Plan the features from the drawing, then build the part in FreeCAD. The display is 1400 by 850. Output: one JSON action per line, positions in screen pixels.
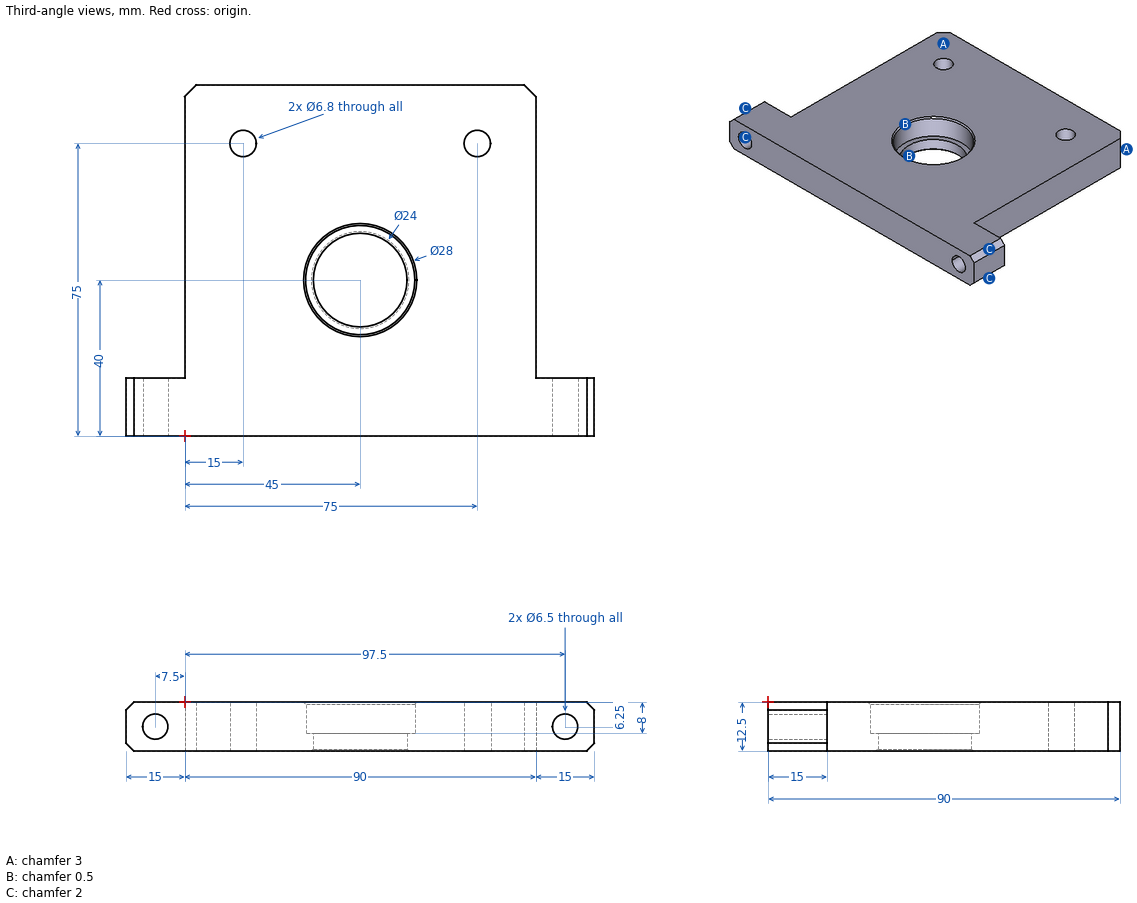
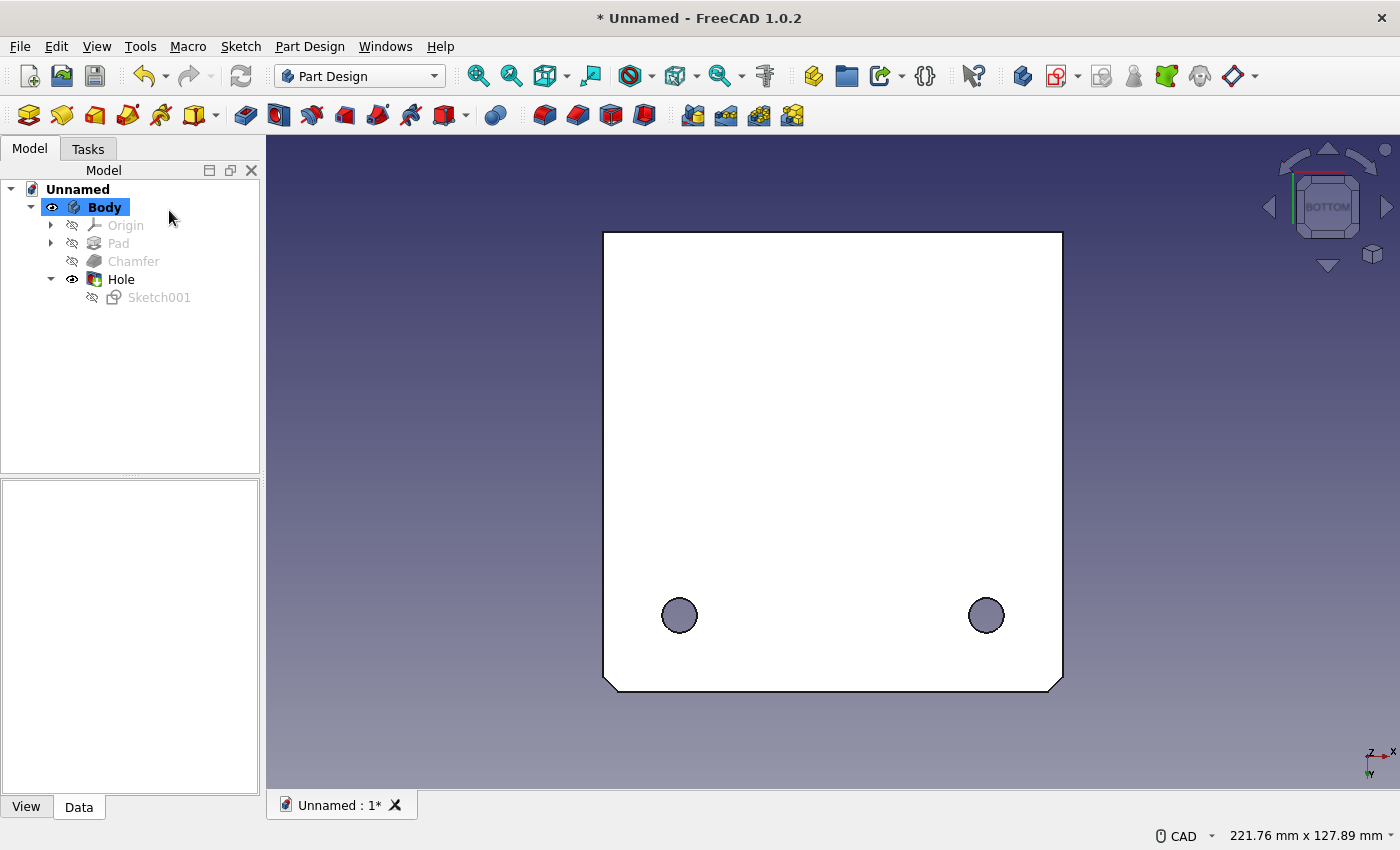
{"action": "left_click", "coordinate": [1056, 76]}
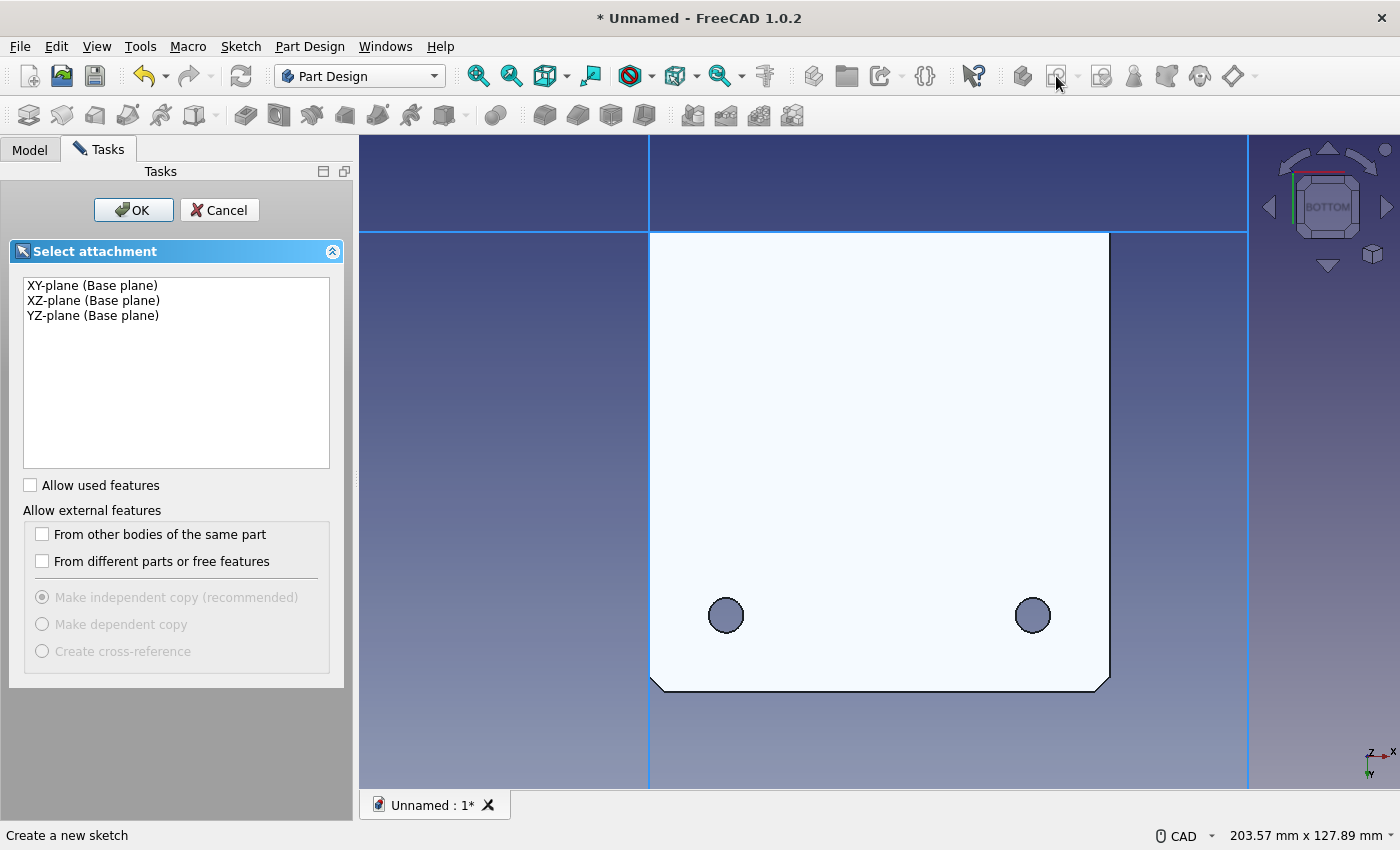
{"action": "left_click", "coordinate": [84, 286]}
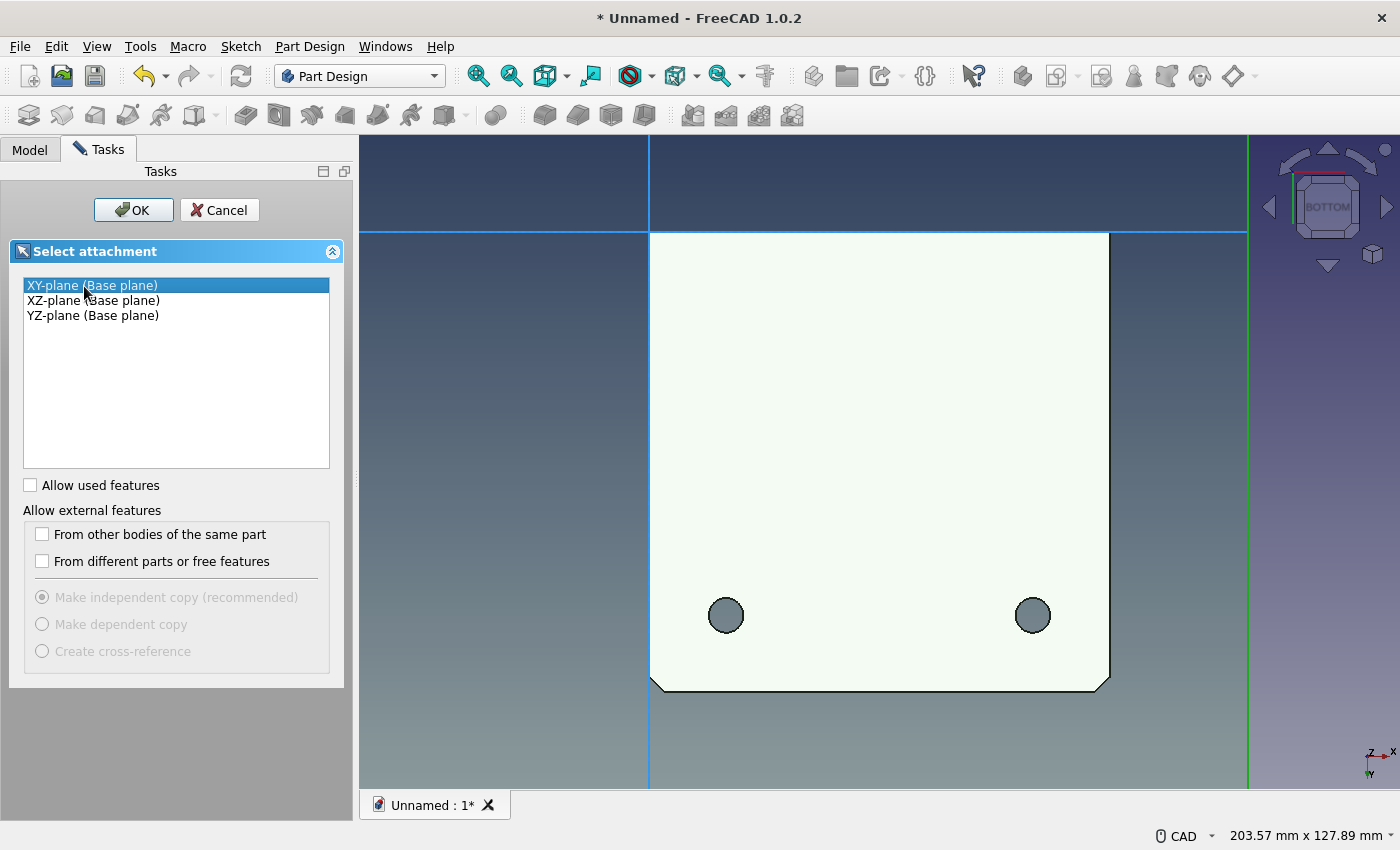
{"action": "left_click", "coordinate": [134, 210]}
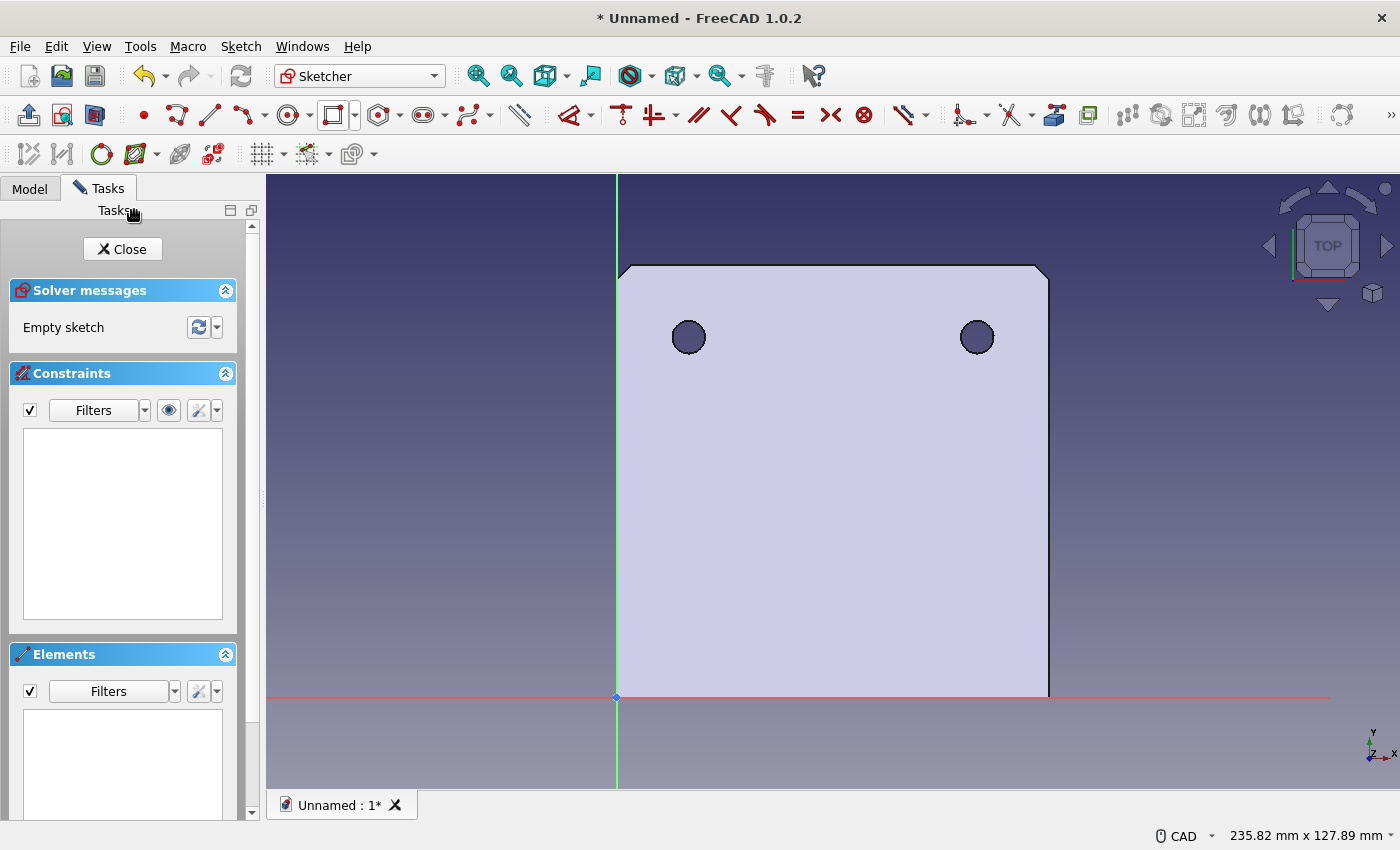
{"action": "scroll", "coordinate": [746, 744], "scroll_direction": "up", "scroll_amount": 2}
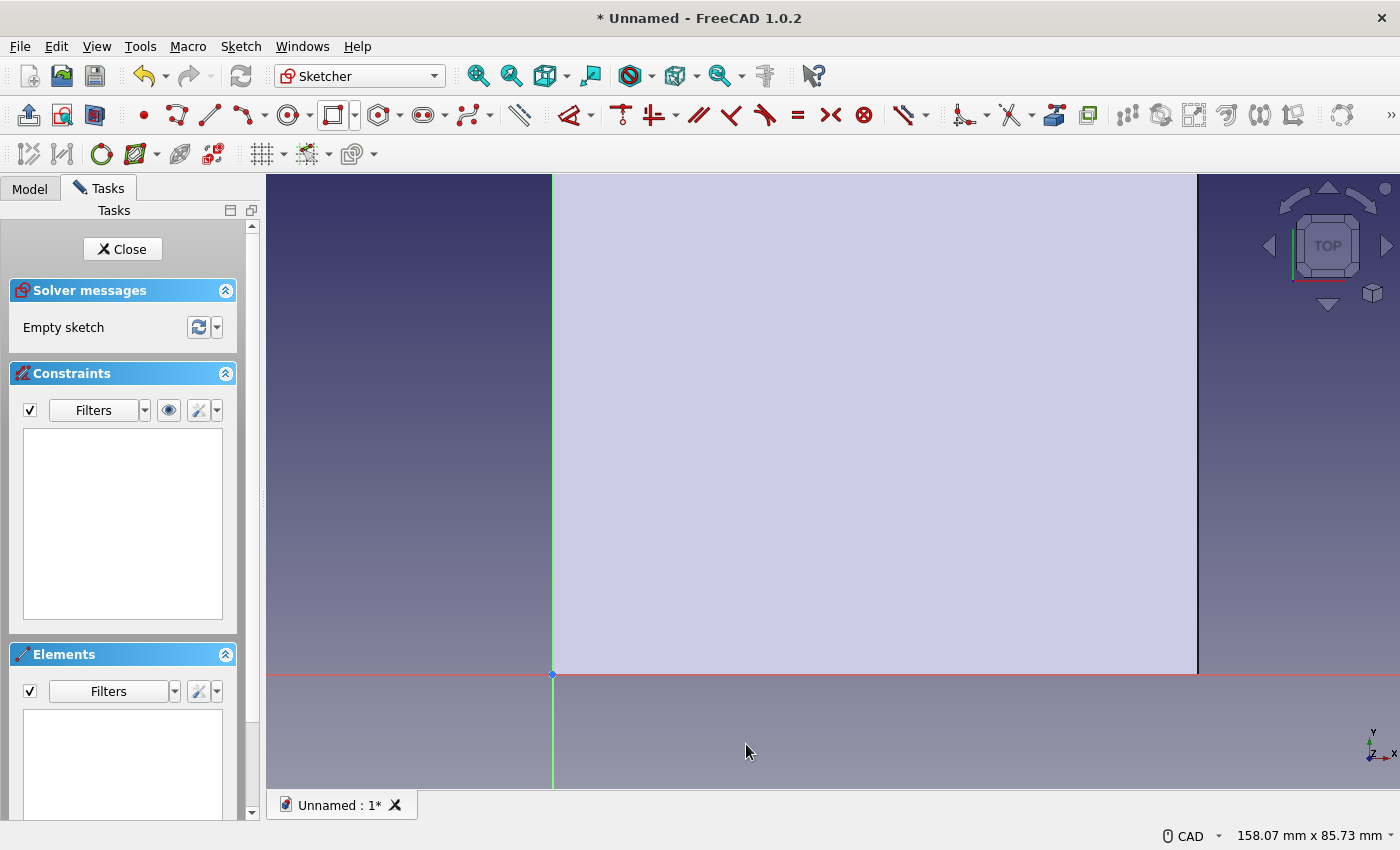
{"action": "left_click", "coordinate": [288, 116]}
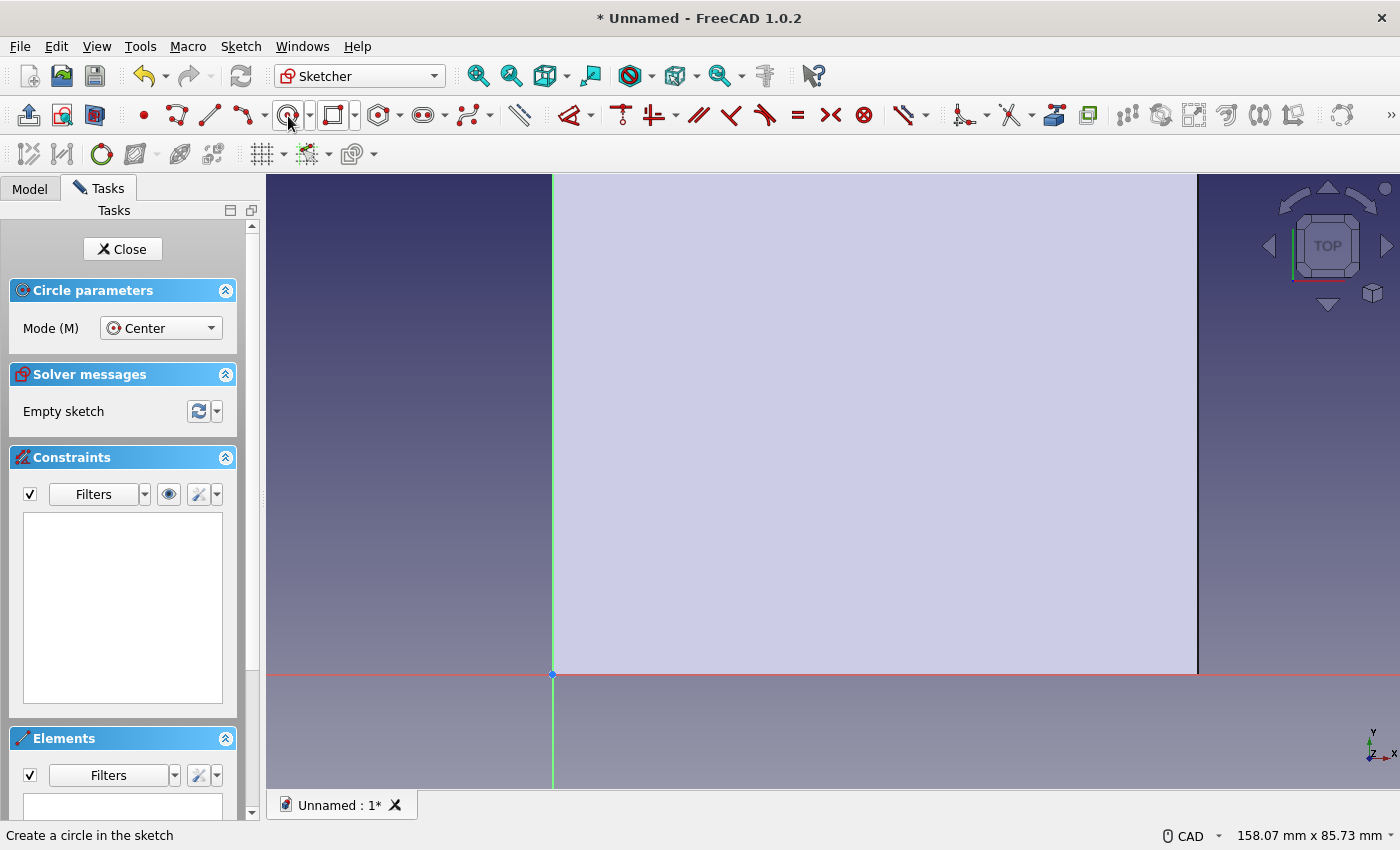
{"action": "left_click", "coordinate": [876, 388]}
{"action": "left_click", "coordinate": [947, 317]}
{"action": "key", "text": "Escape"}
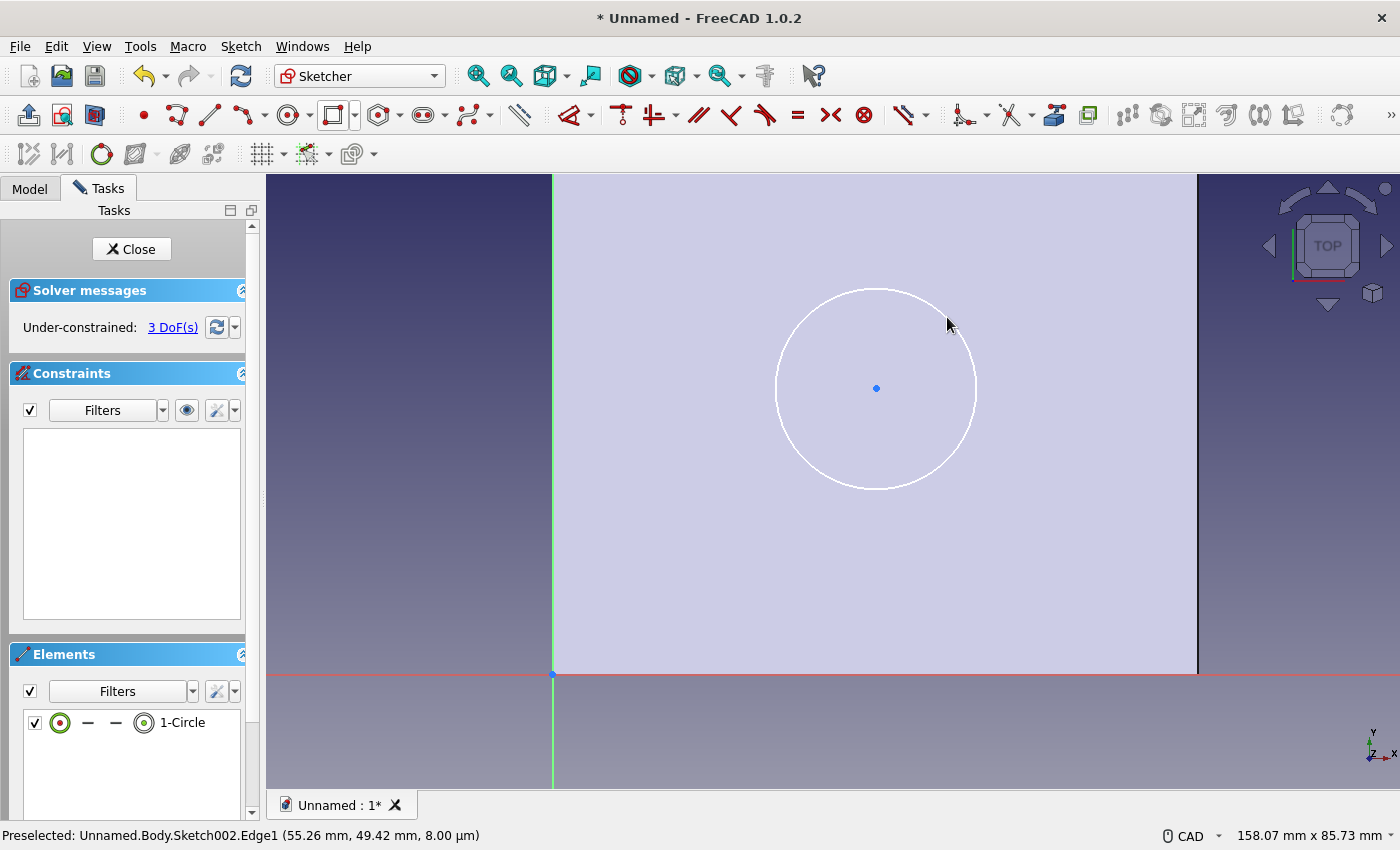
{"action": "left_click", "coordinate": [568, 116]}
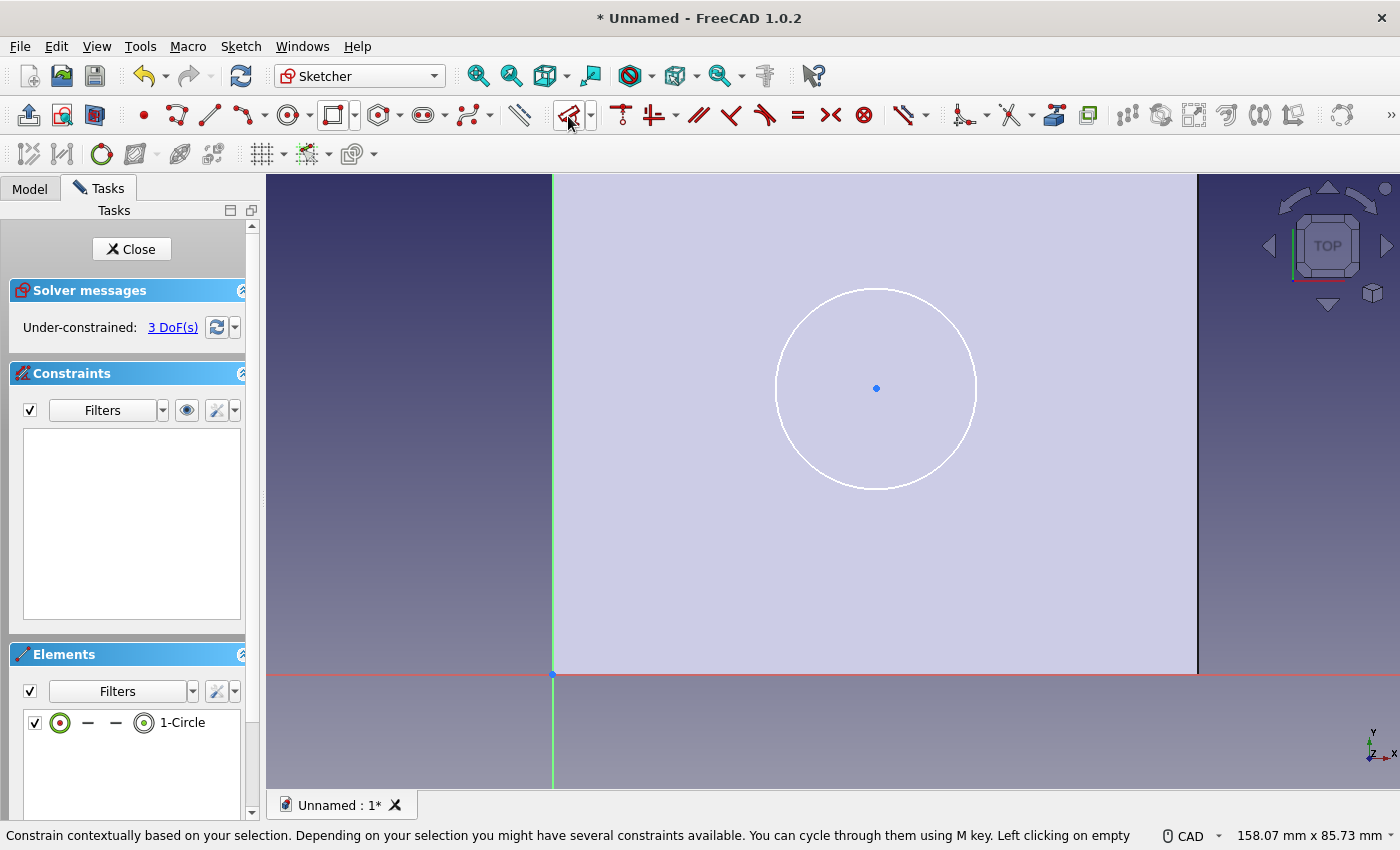
{"action": "left_click", "coordinate": [947, 318]}
{"action": "left_click", "coordinate": [970, 295]}